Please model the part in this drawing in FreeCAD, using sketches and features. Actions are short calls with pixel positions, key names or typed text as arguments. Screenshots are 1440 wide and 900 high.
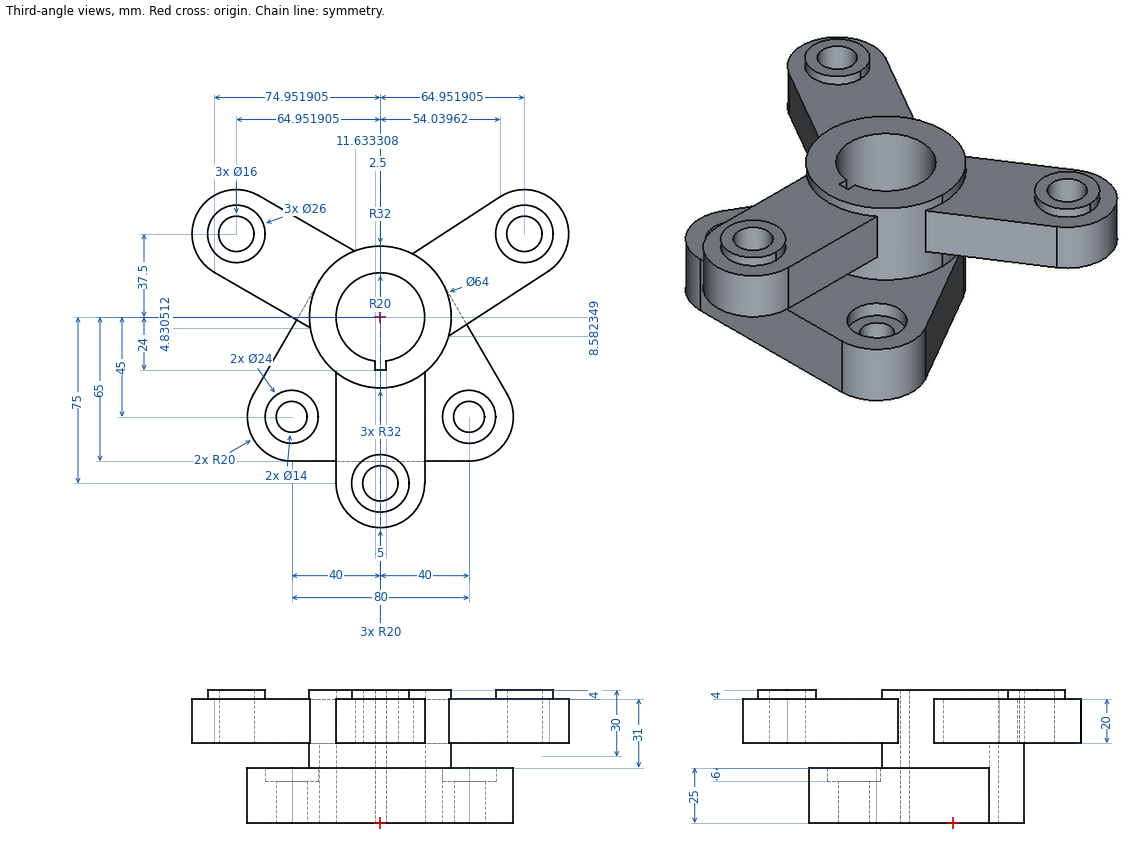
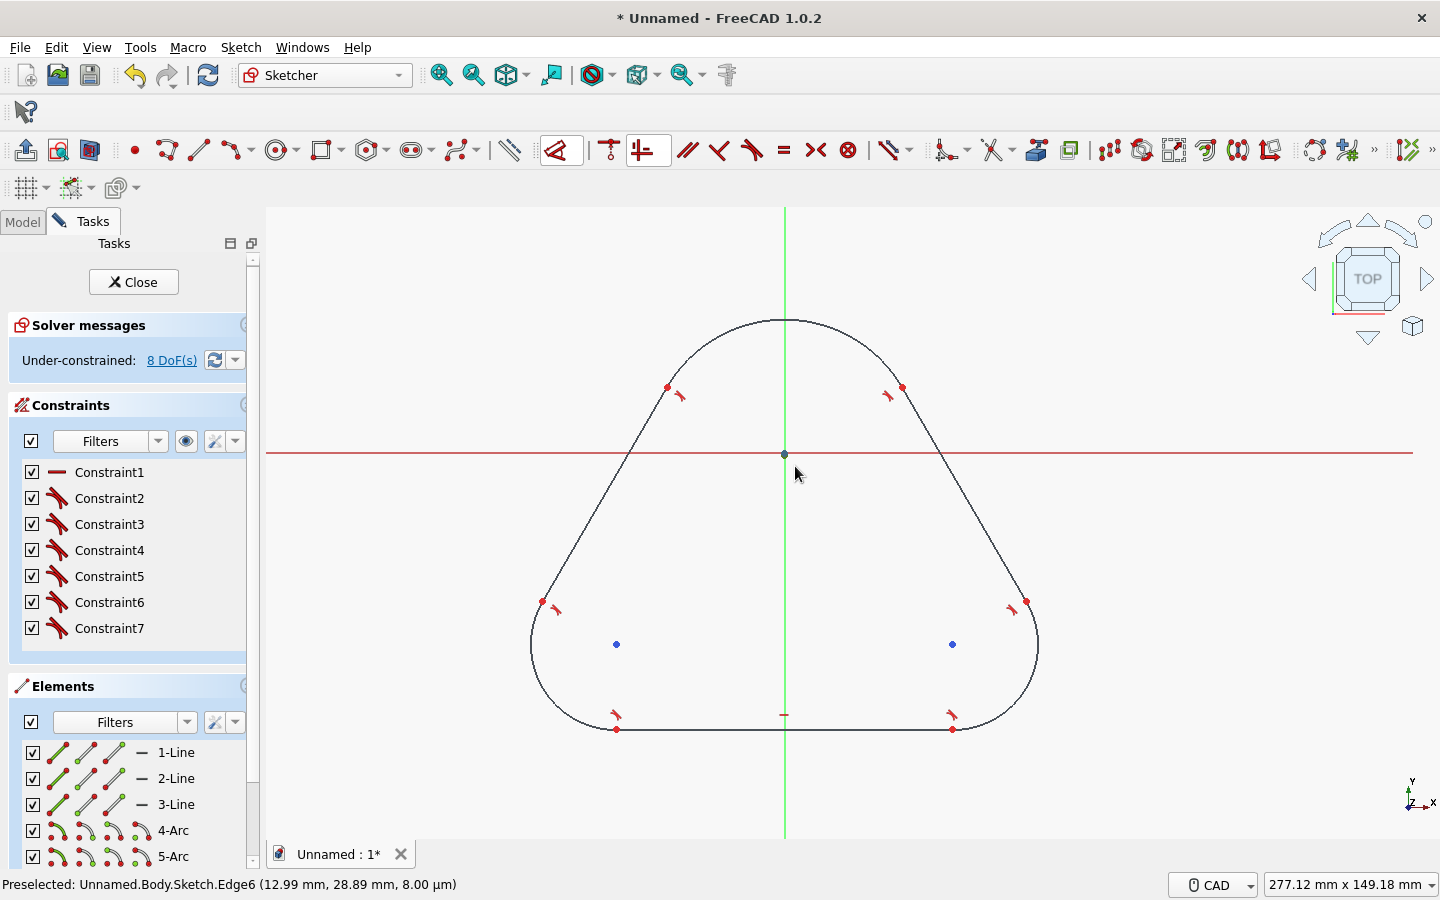
click(610, 150)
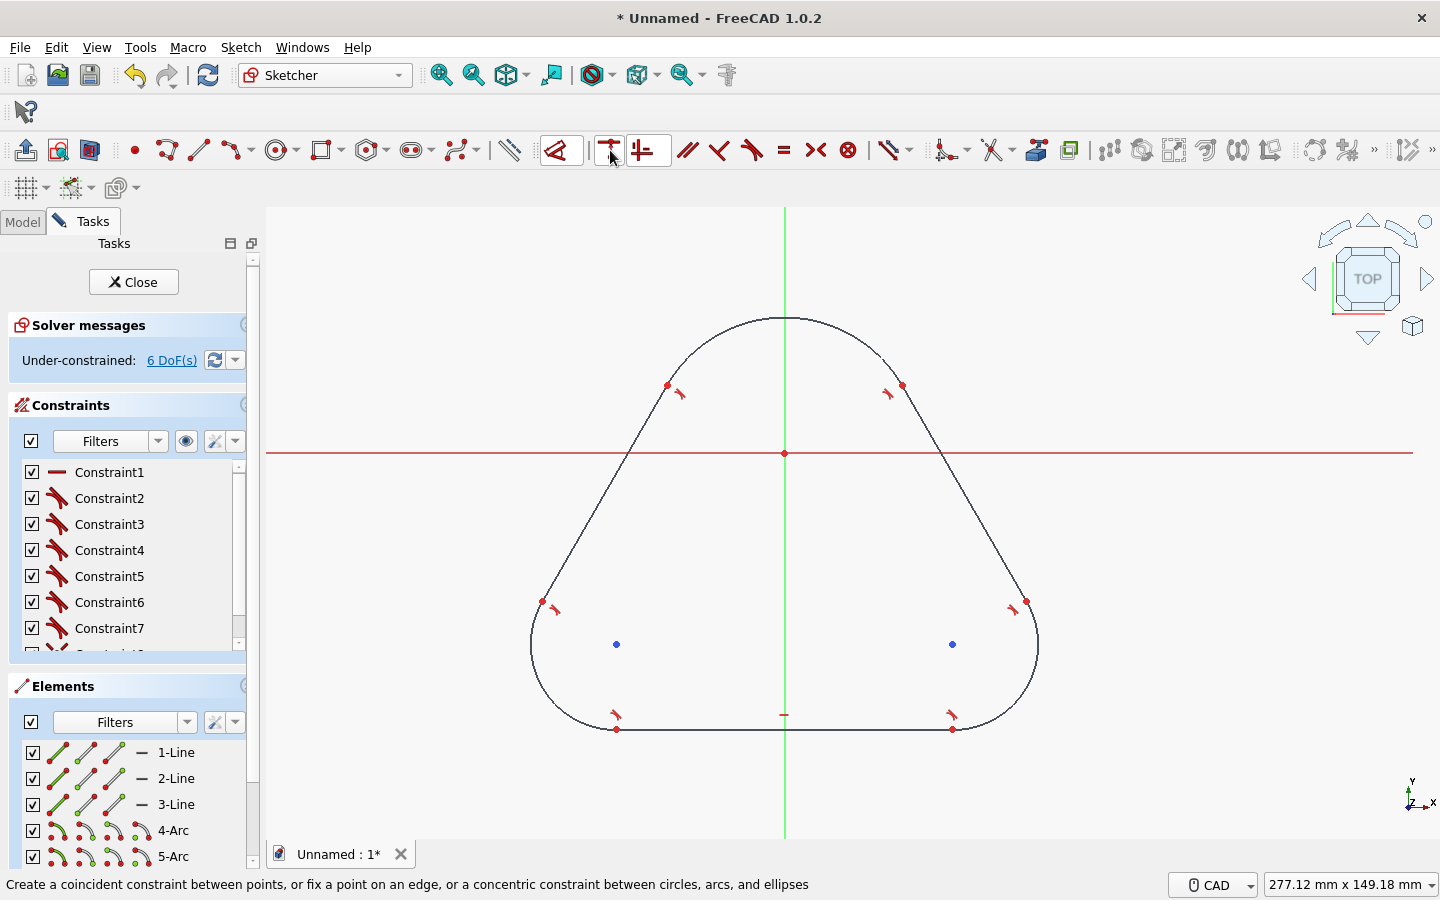
click(531, 654)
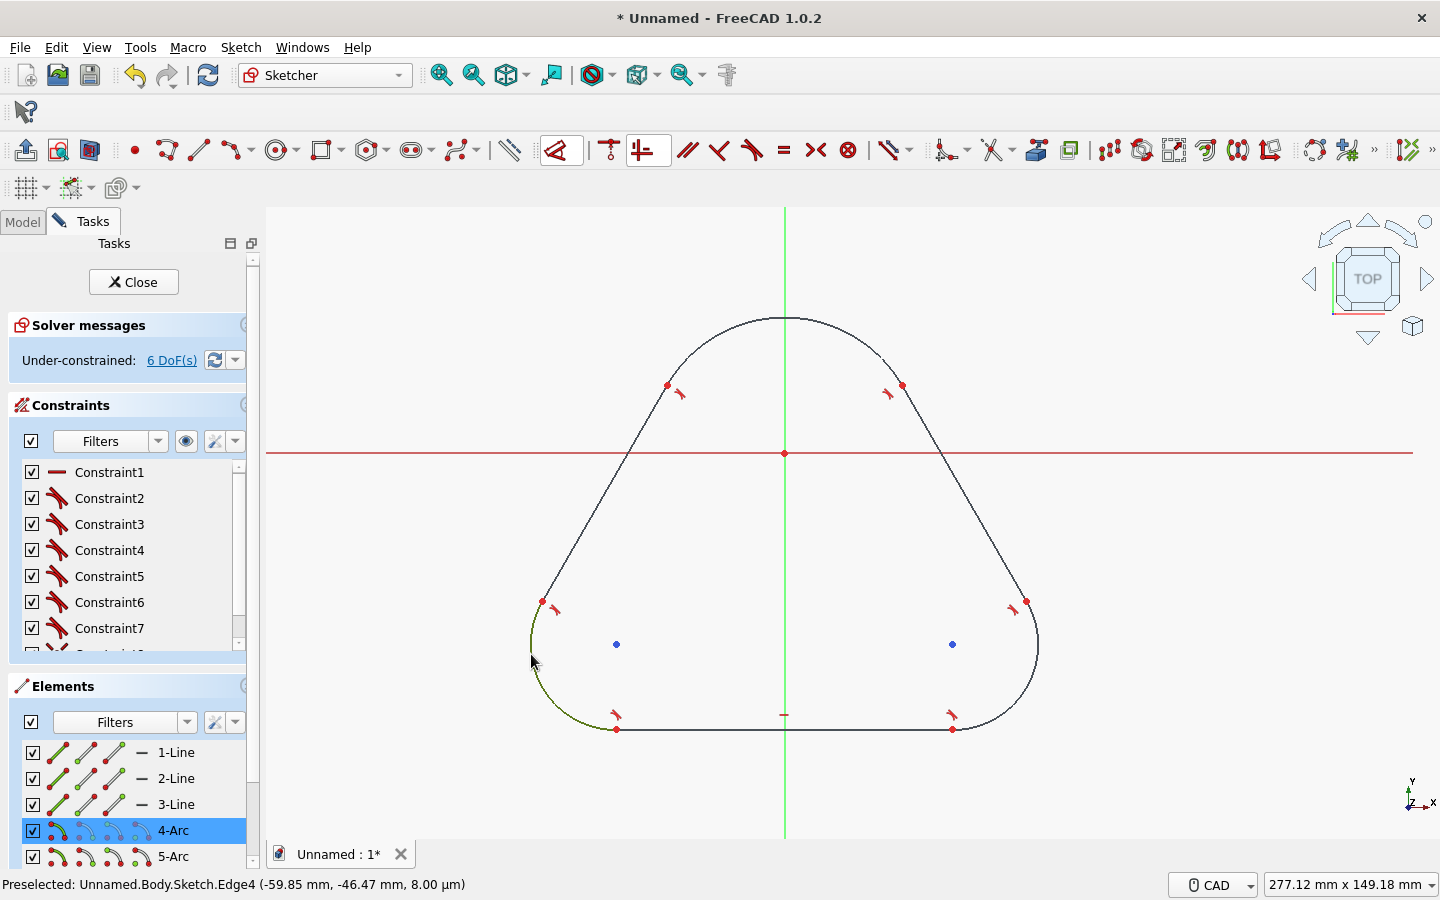
click(1003, 714)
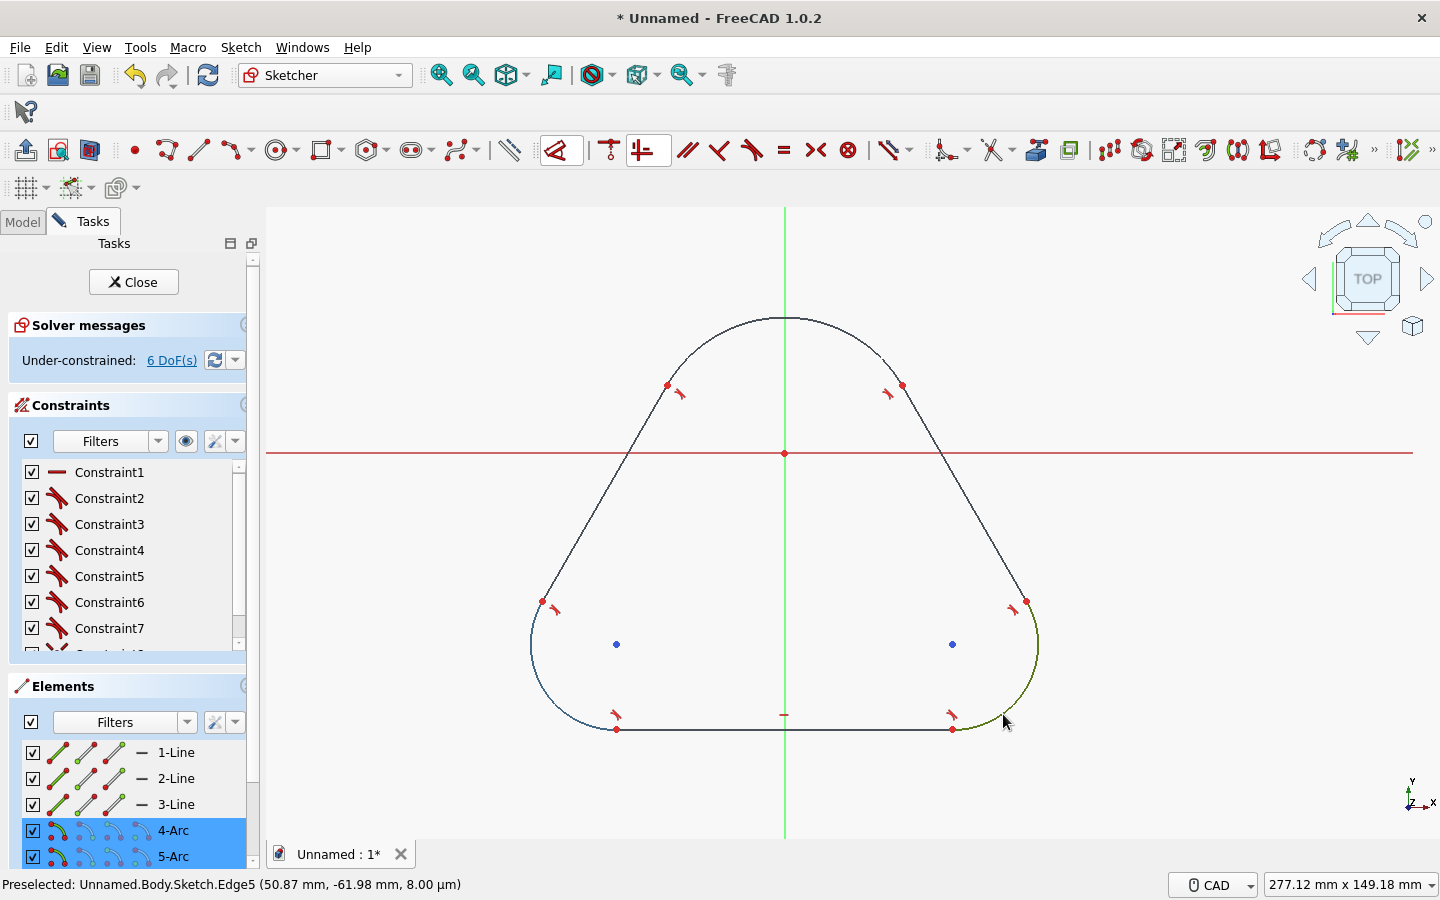
click(784, 150)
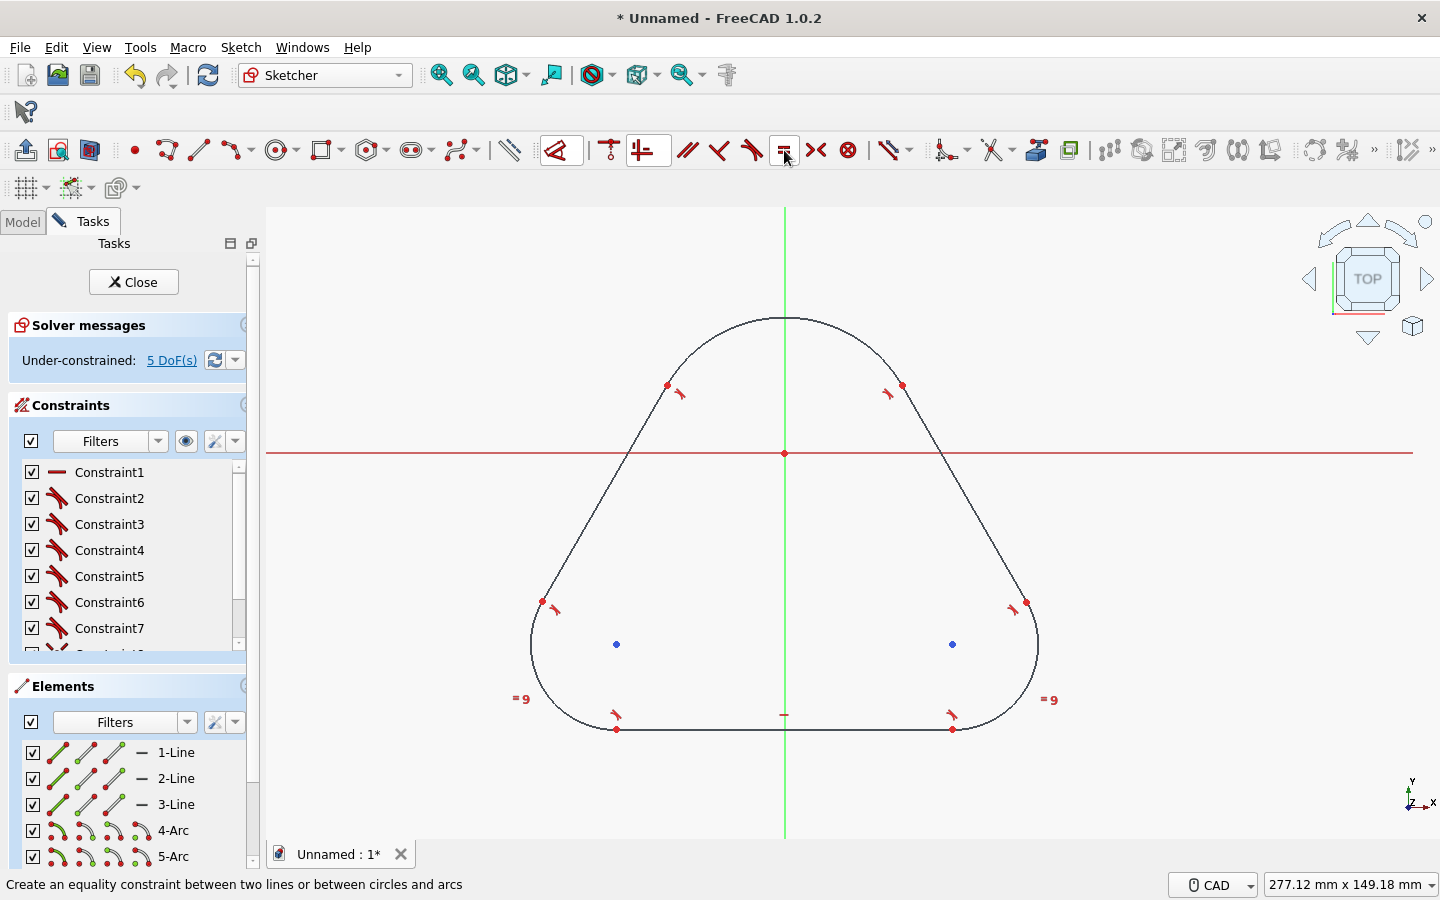
key(d)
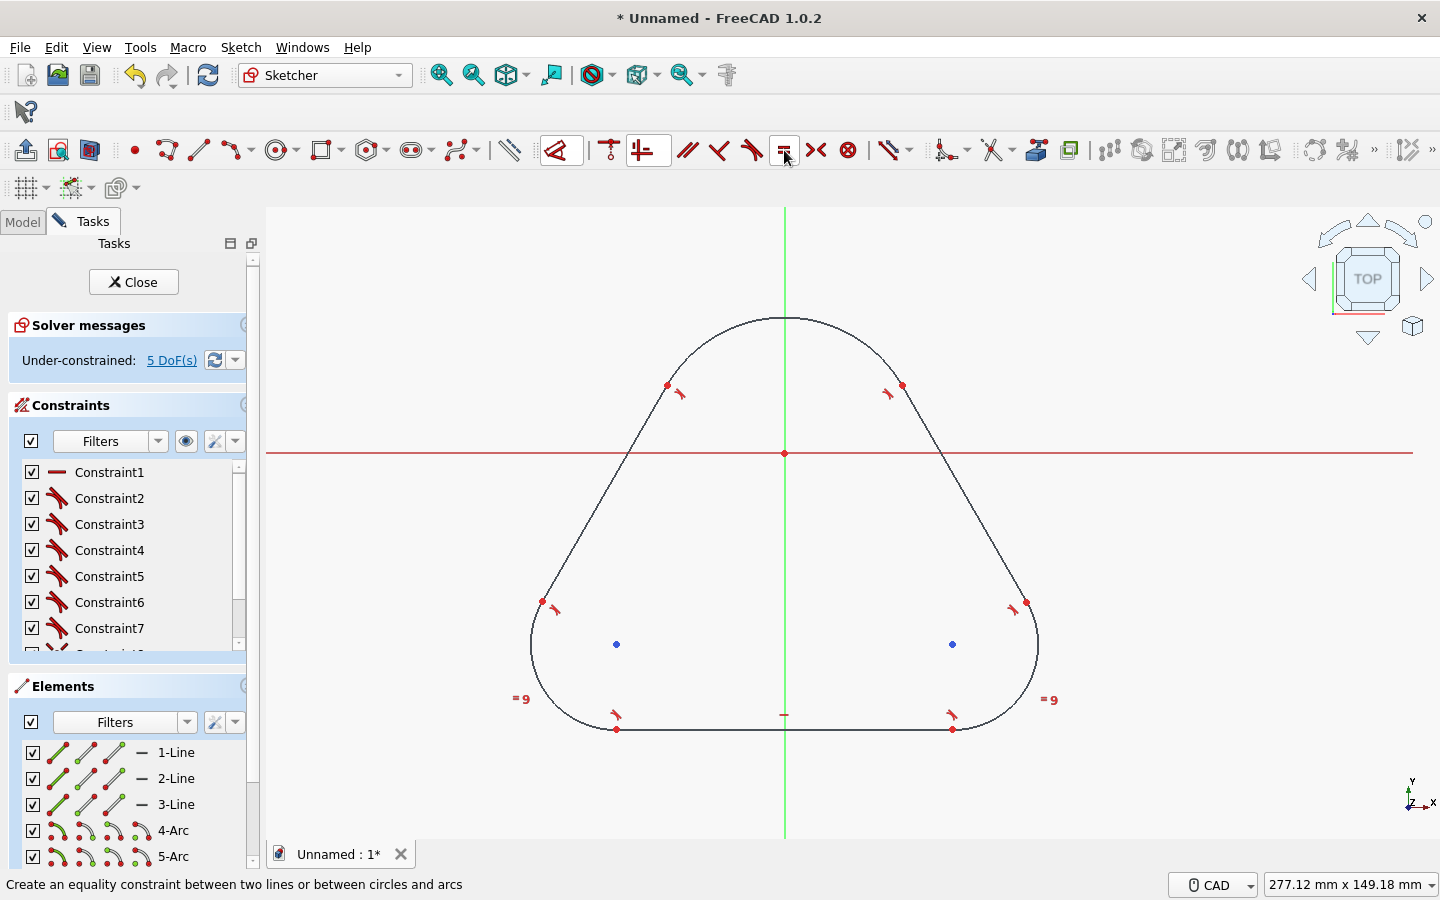
click(531, 654)
click(499, 657)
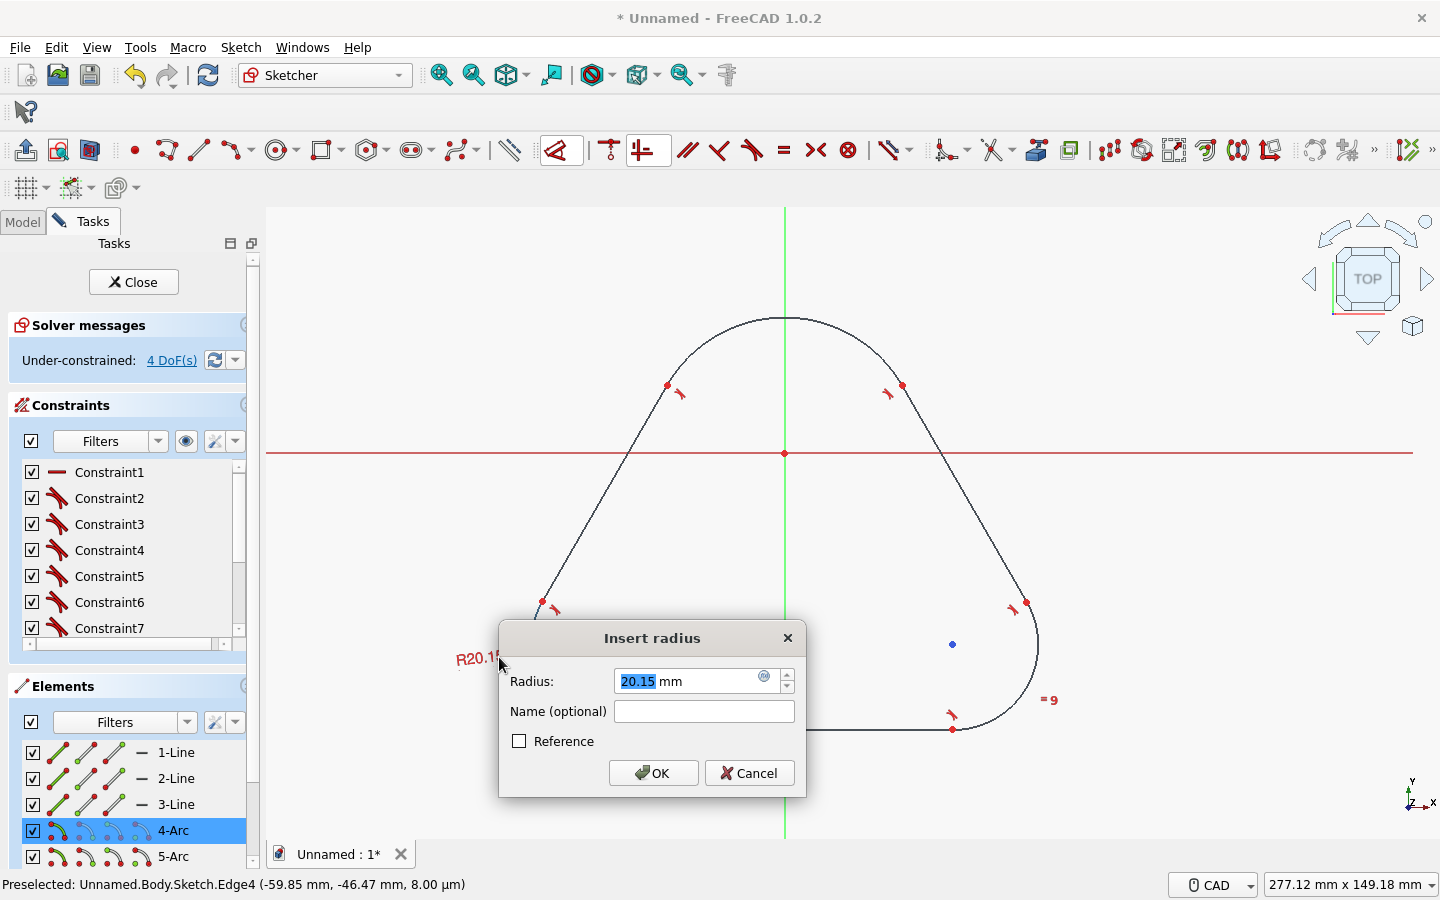
text(20)
key(Return)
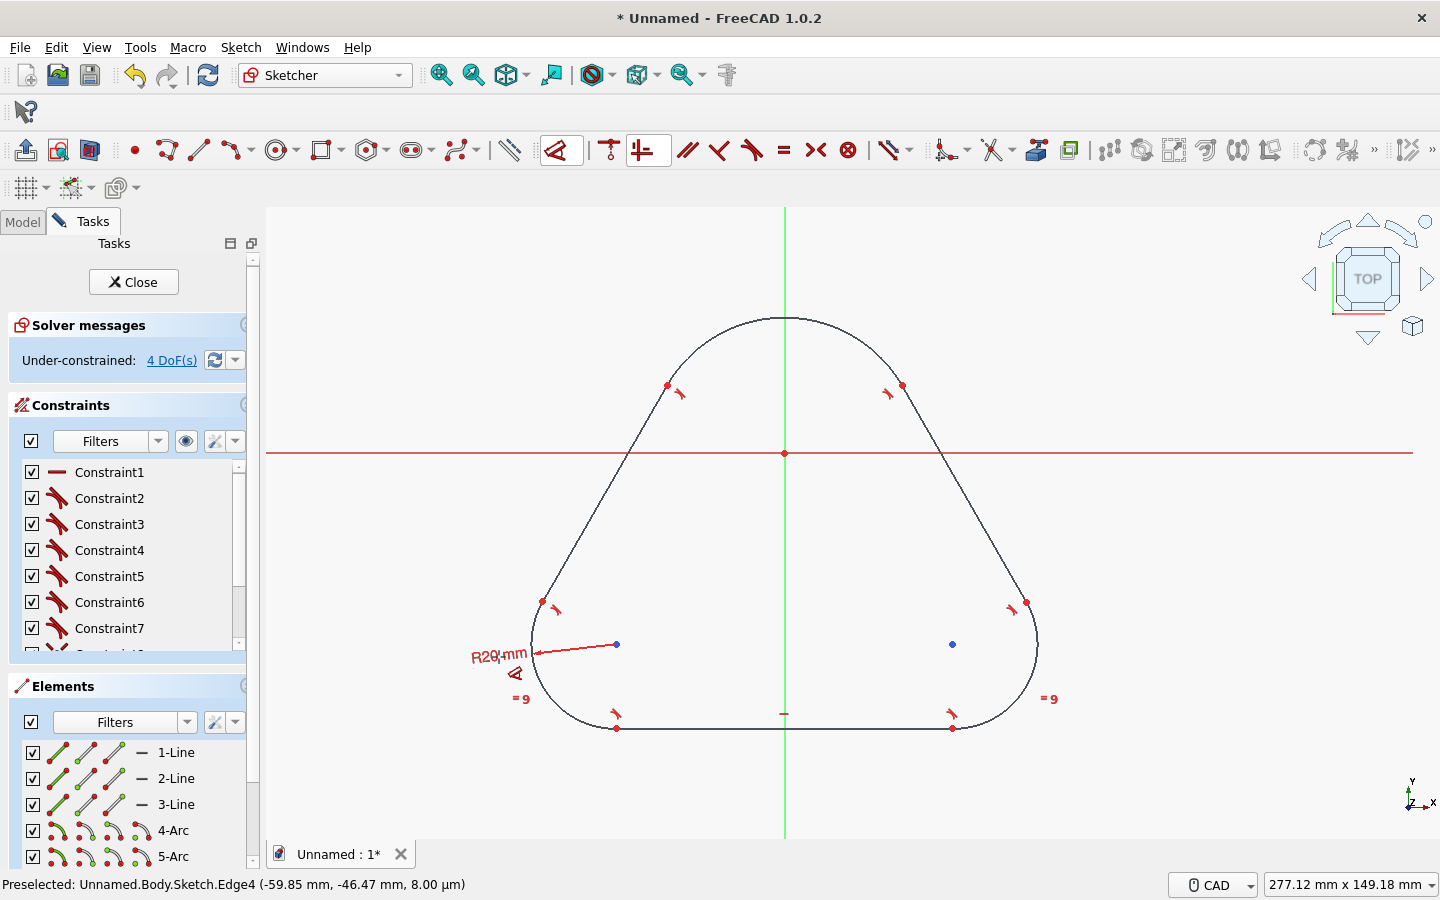
click(840, 329)
click(853, 300)